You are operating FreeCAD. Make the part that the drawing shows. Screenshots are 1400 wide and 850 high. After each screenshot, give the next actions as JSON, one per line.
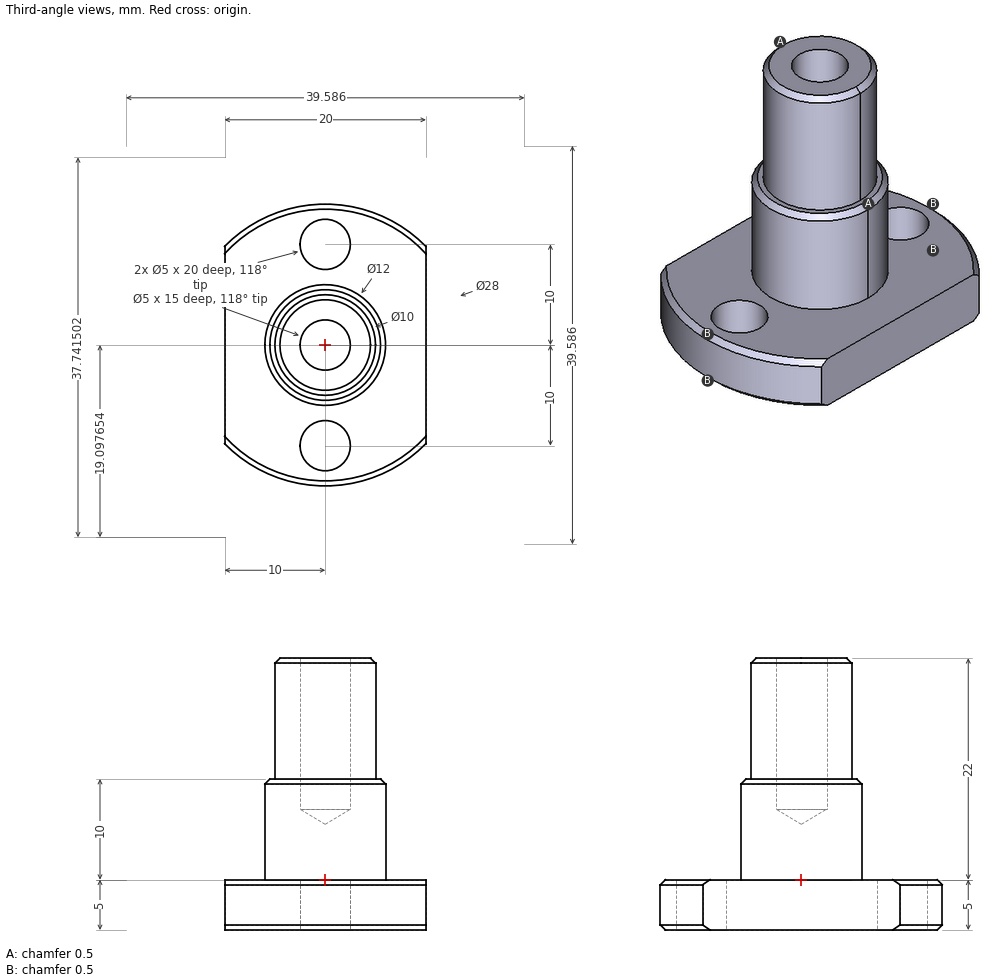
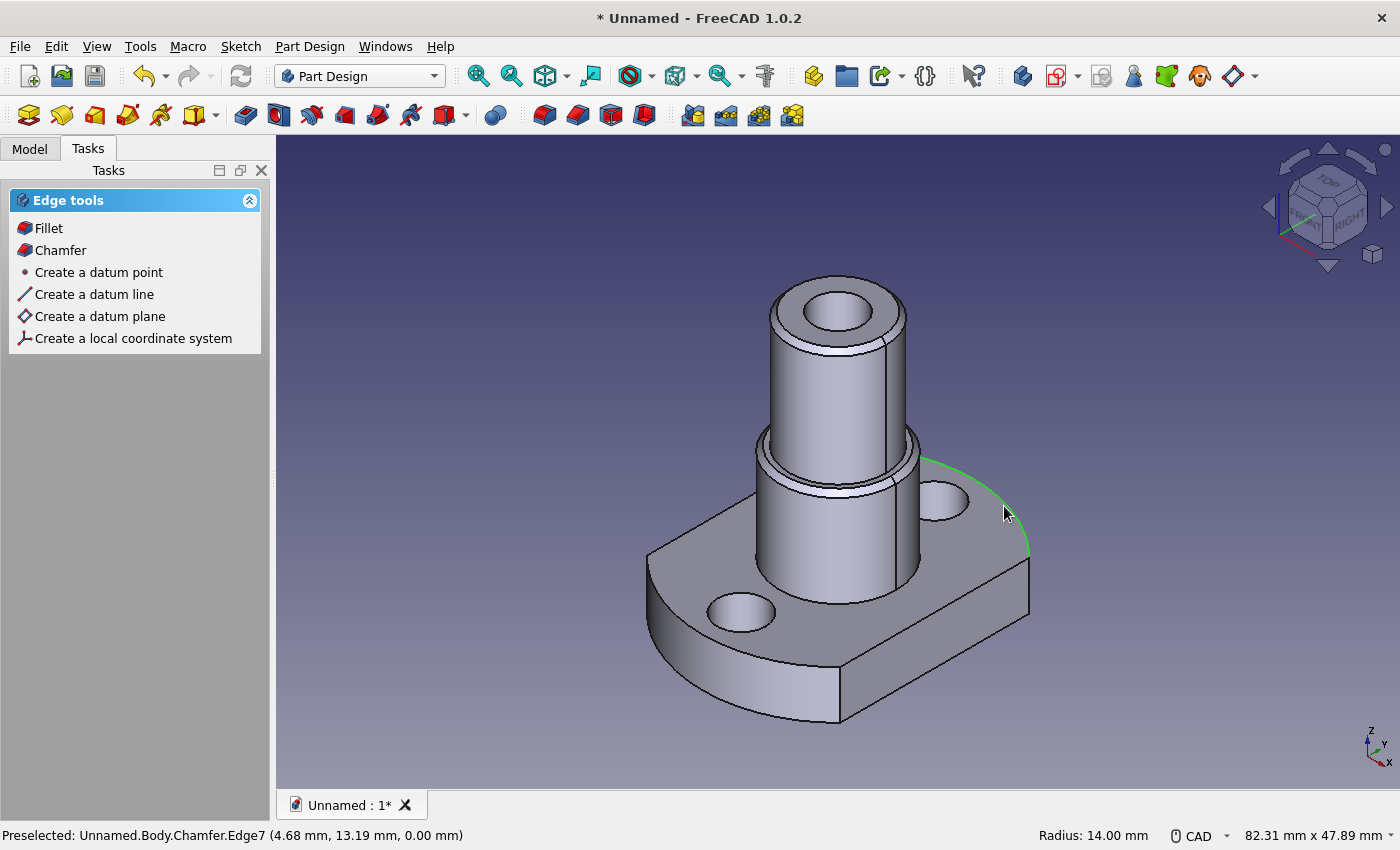
{"action": "left_click", "coordinate": [703, 634], "text": "ctrl"}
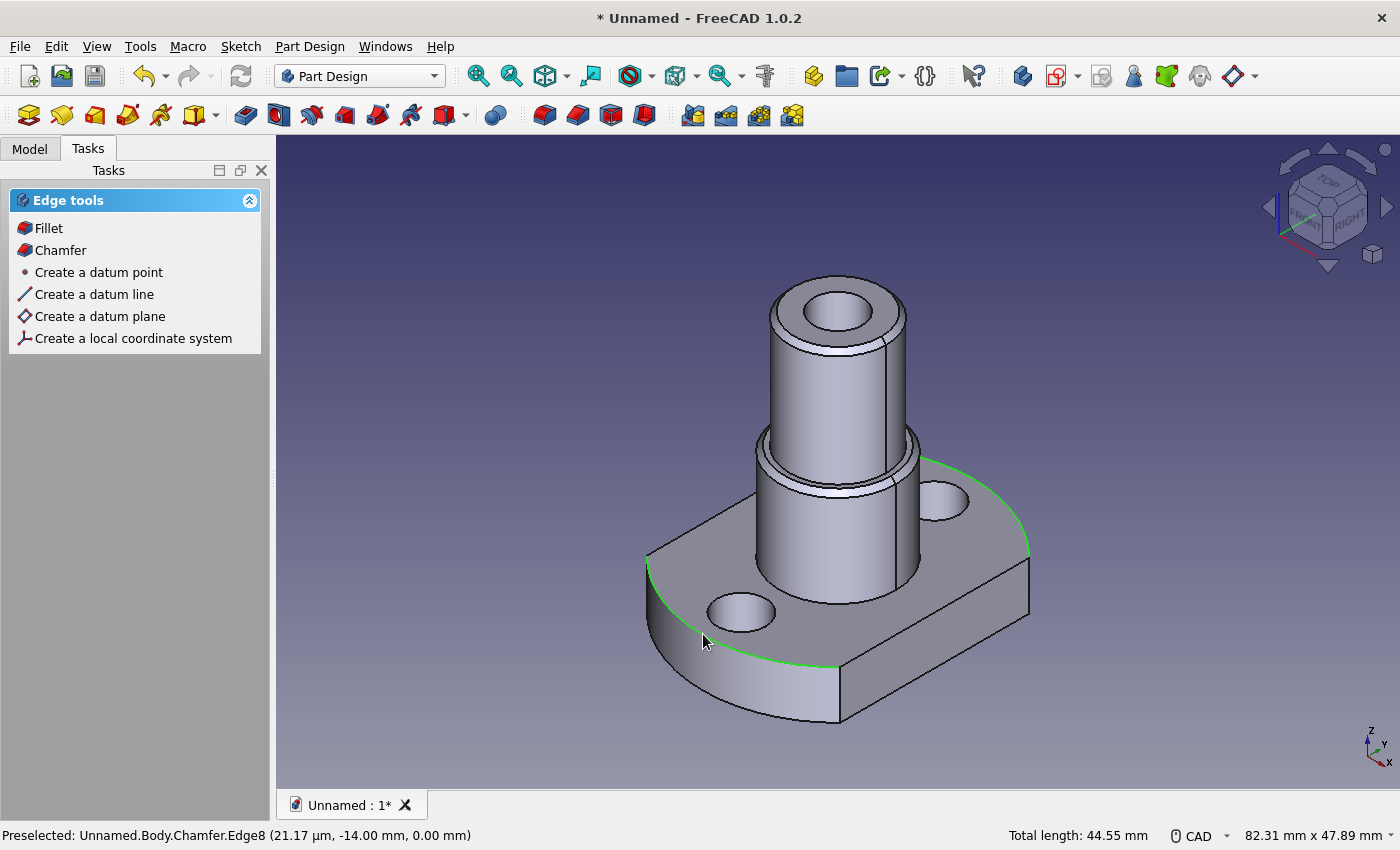
{"action": "key", "text": "2"}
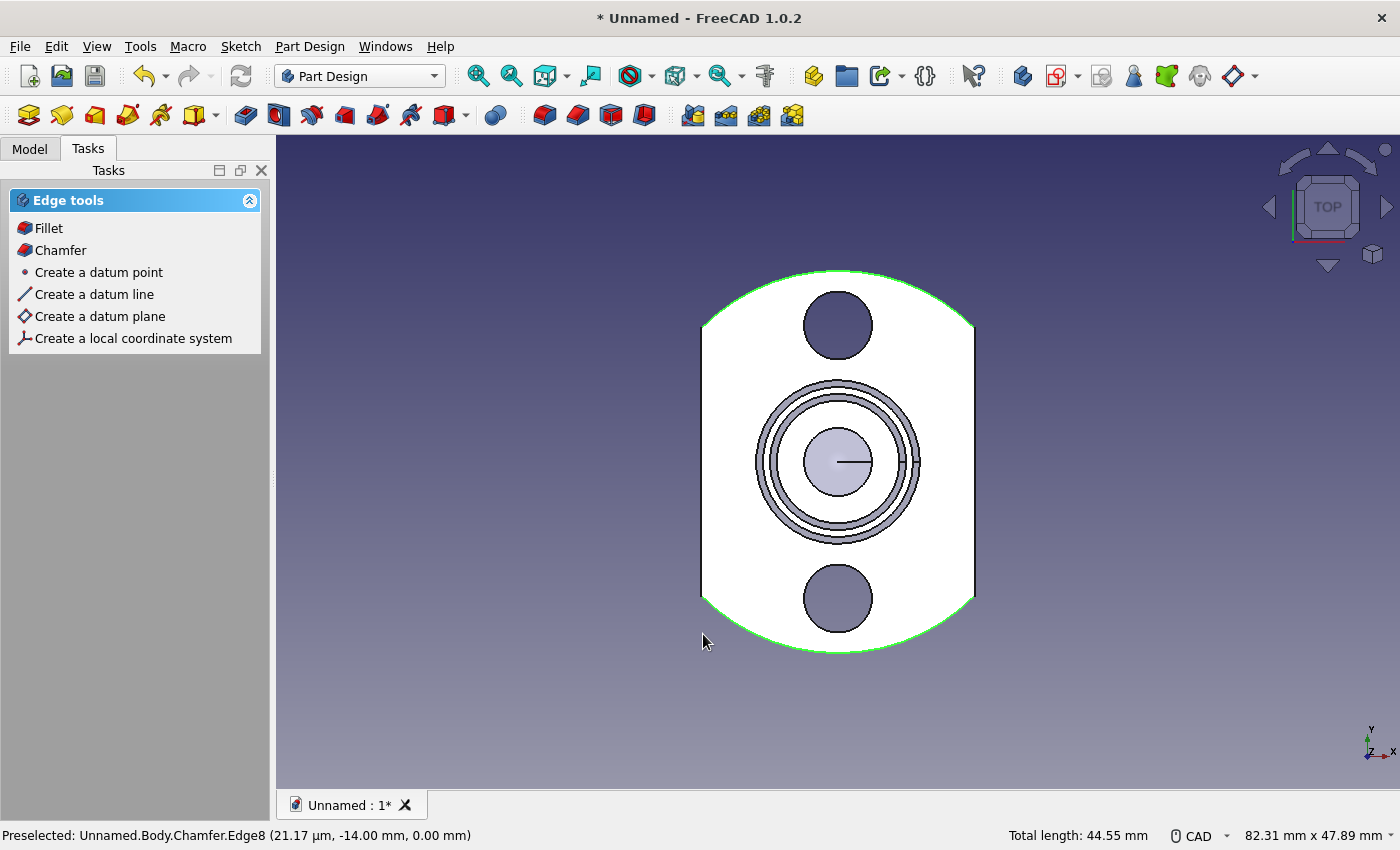
{"action": "key", "text": "0"}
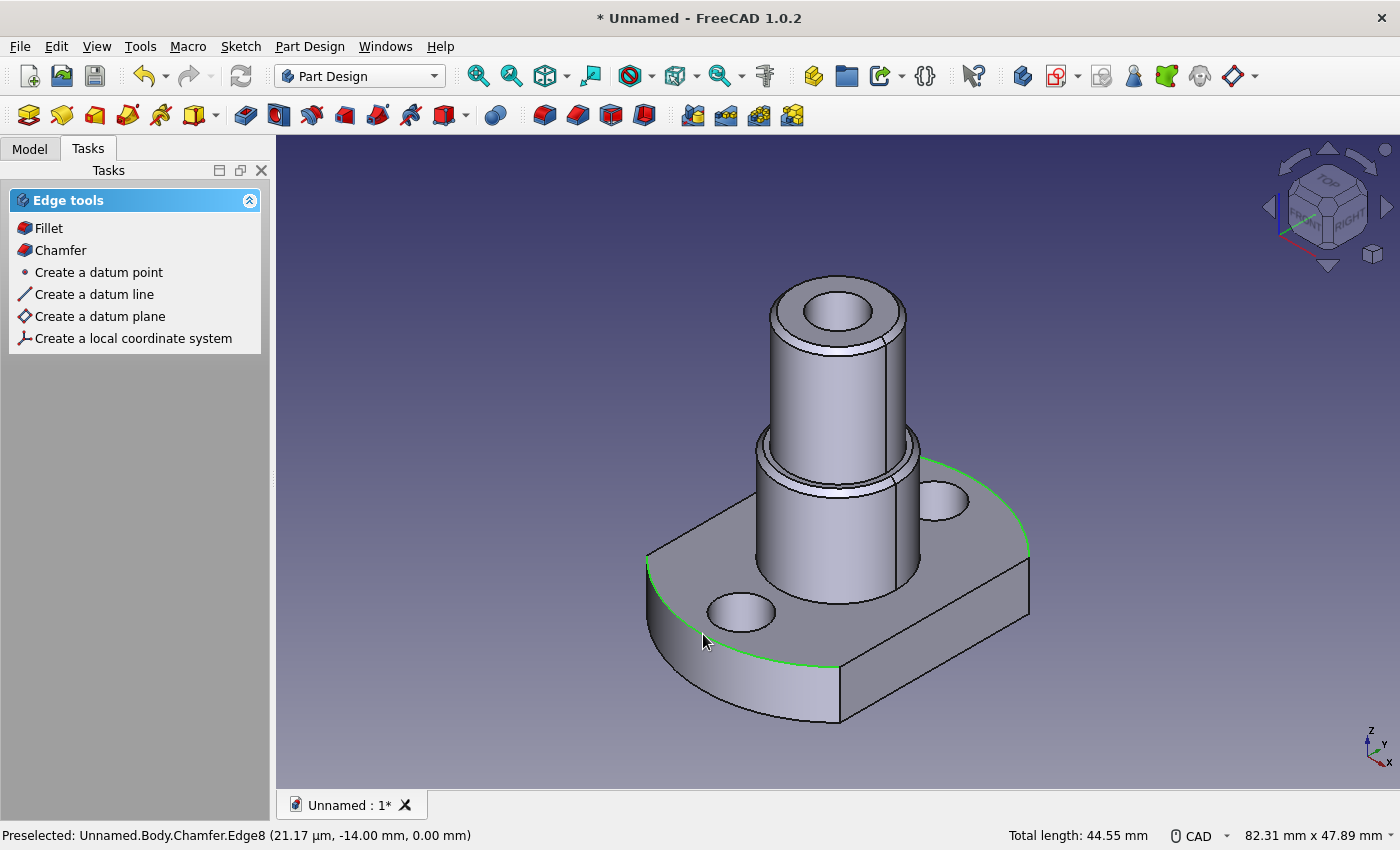
{"action": "key", "text": "1"}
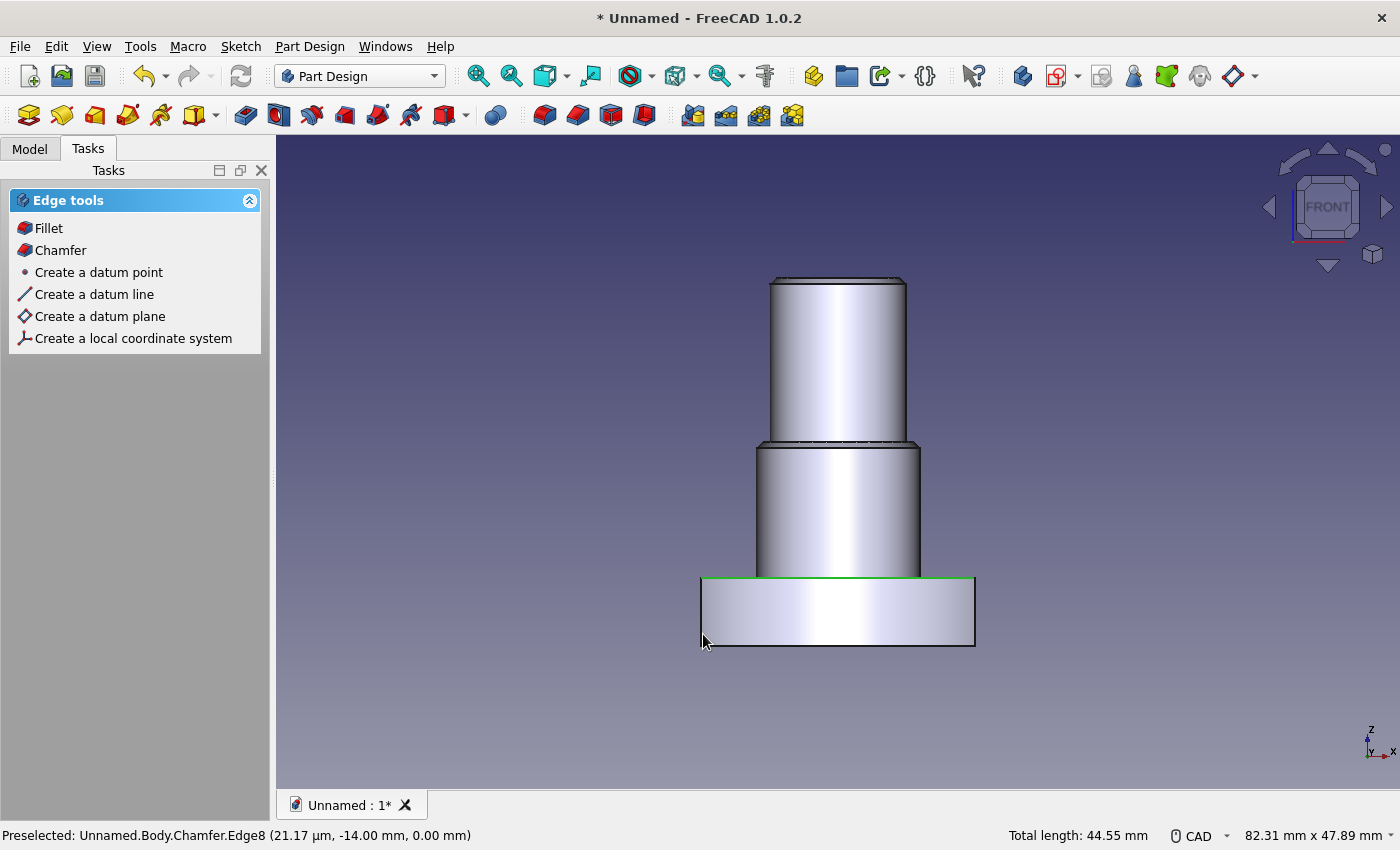
{"action": "left_click", "coordinate": [838, 645], "text": "ctrl"}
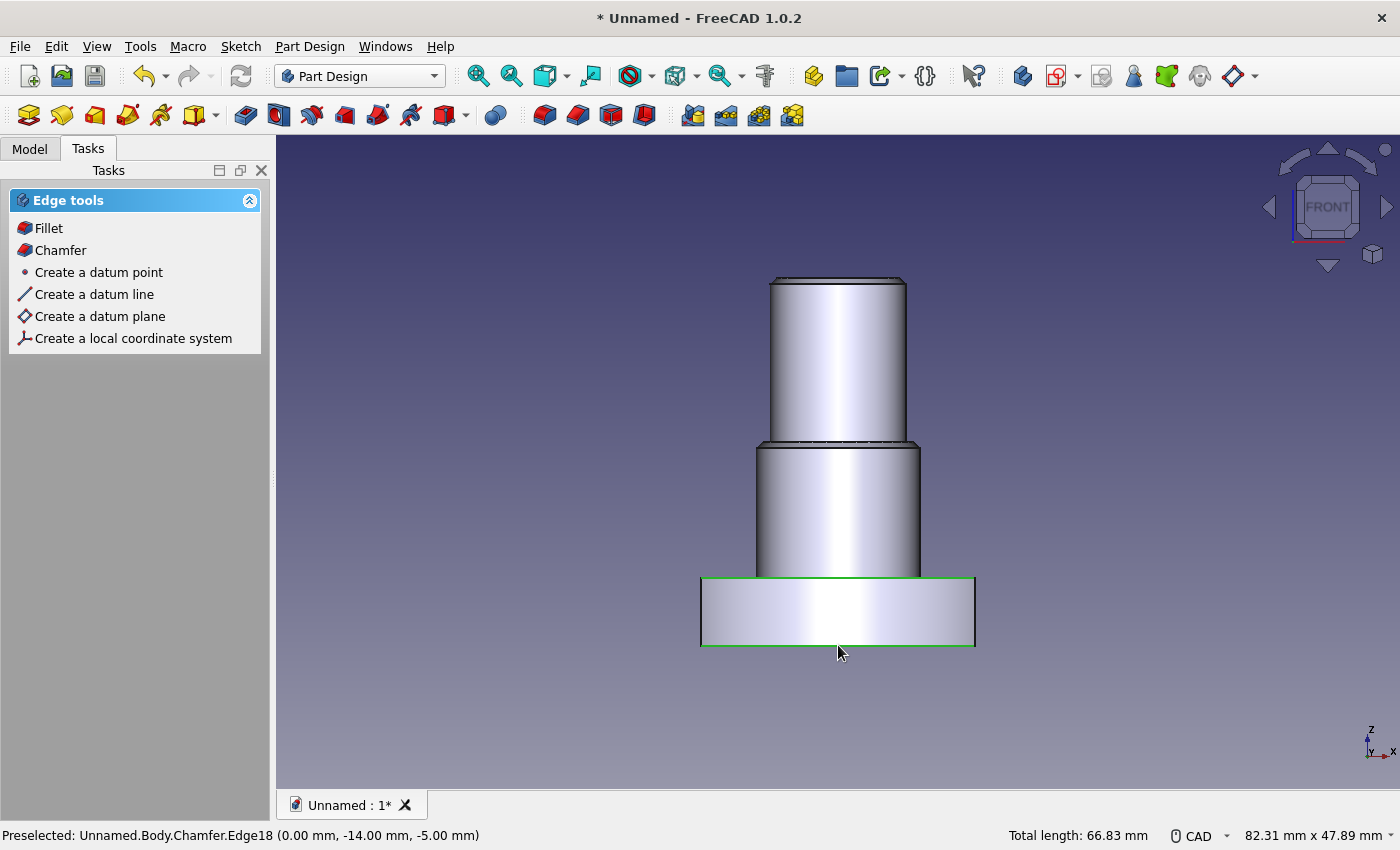
{"action": "key", "text": "3"}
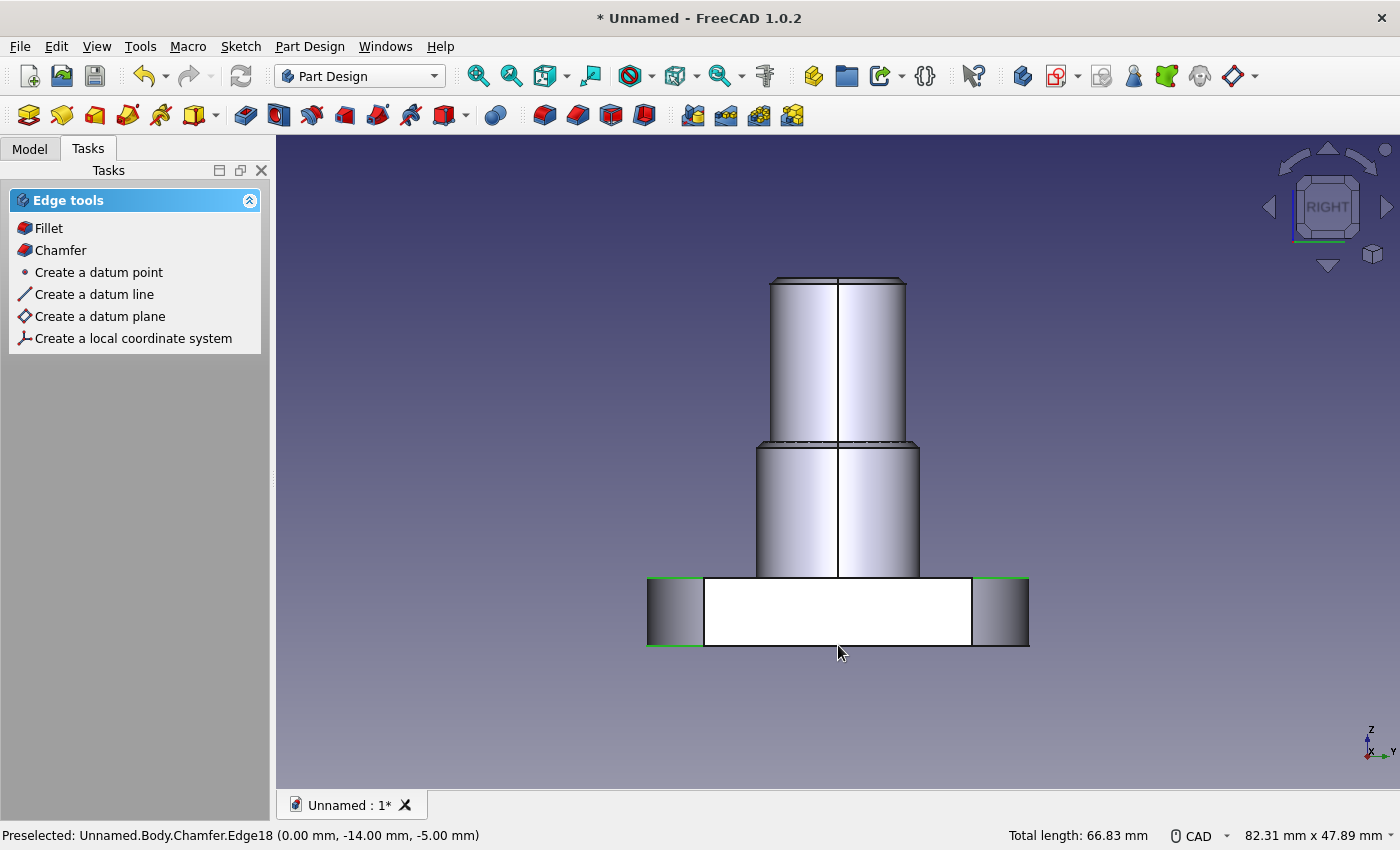
{"action": "left_click", "coordinate": [1027, 645], "text": "ctrl"}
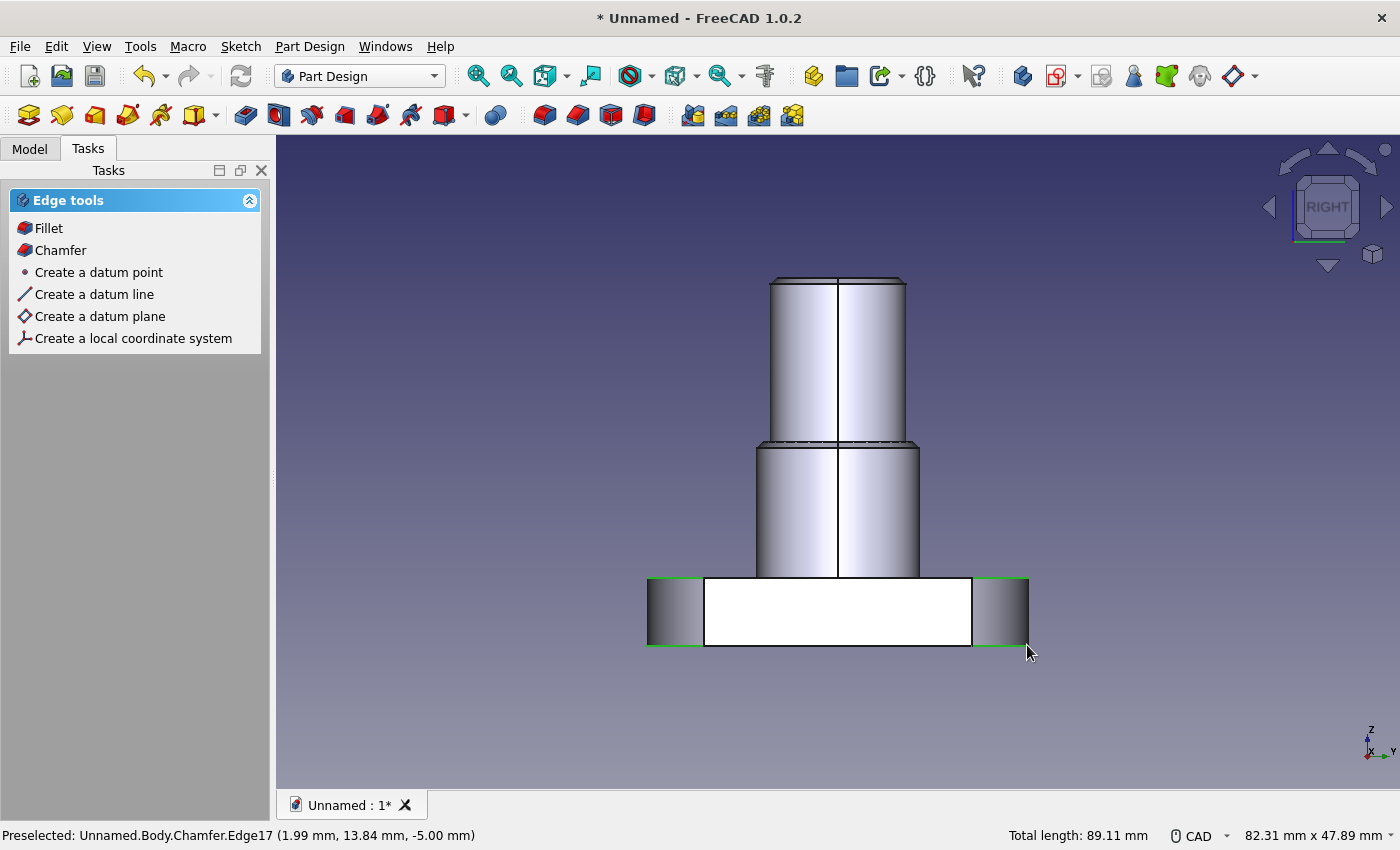
{"action": "left_click", "coordinate": [578, 116]}